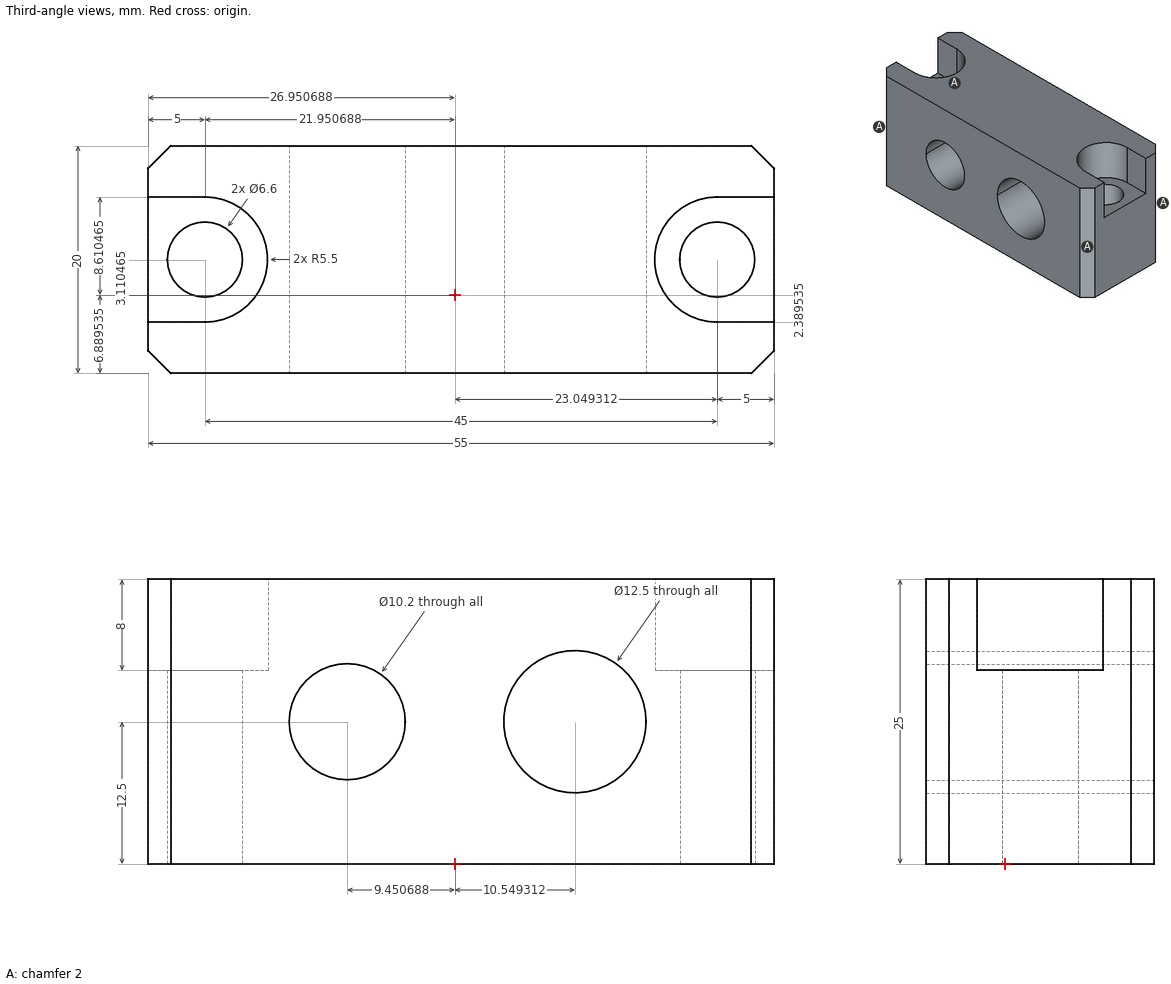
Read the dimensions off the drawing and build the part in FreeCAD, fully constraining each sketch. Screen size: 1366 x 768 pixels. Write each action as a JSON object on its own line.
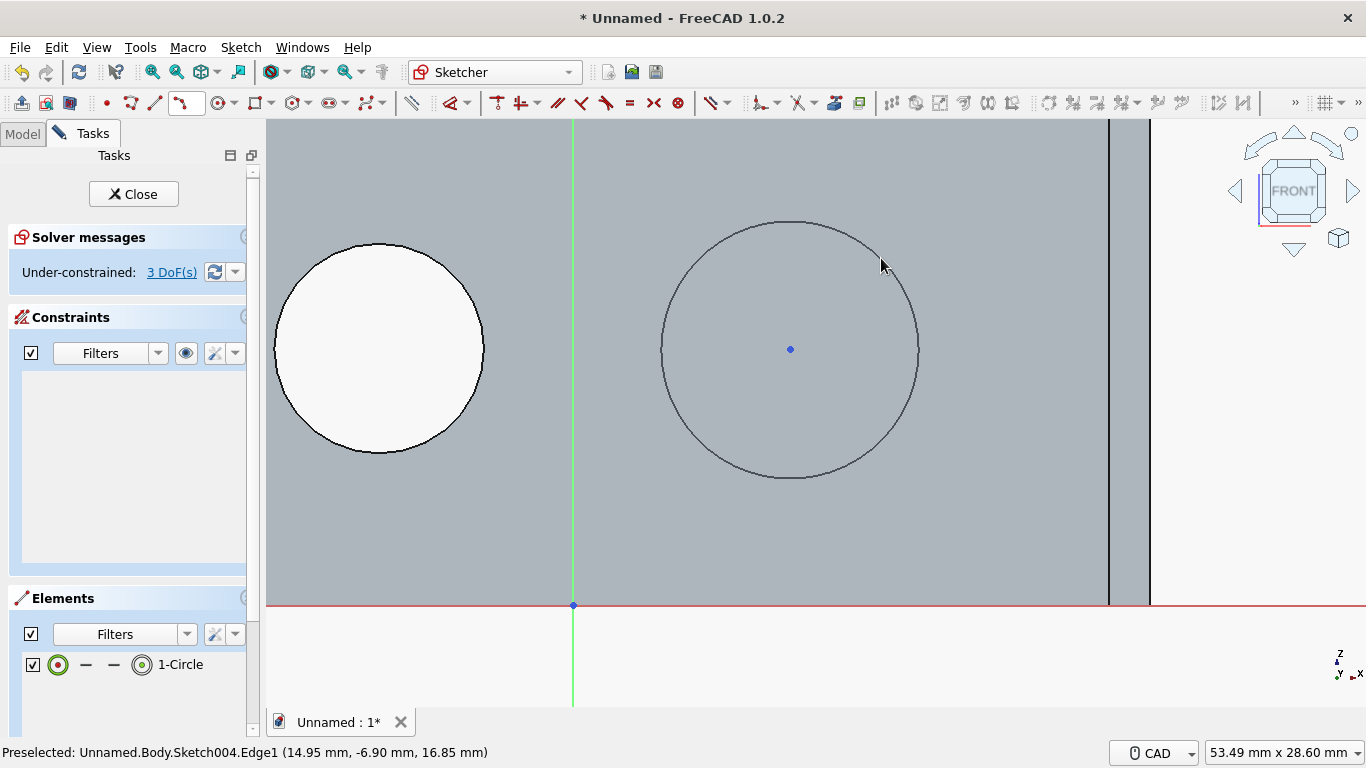
{"action": "key", "text": "d"}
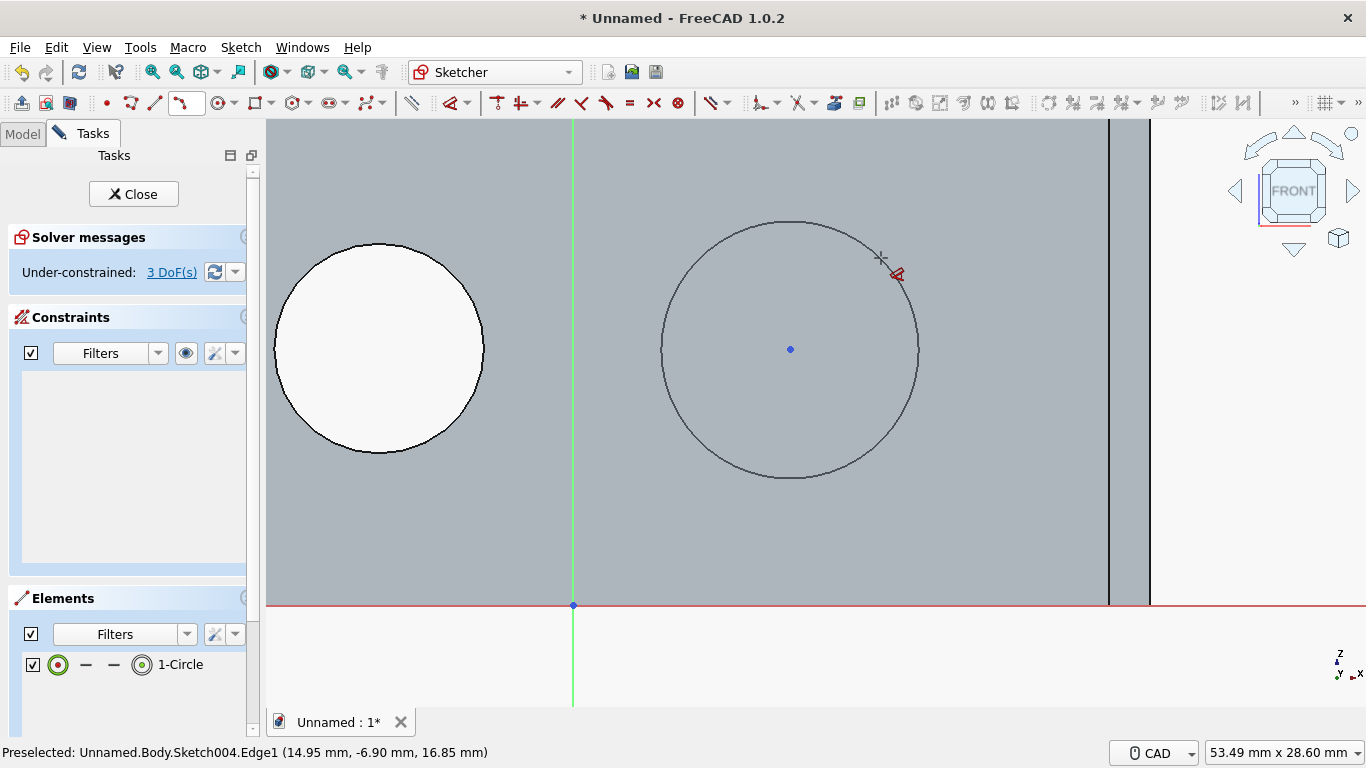
{"action": "left_click", "coordinate": [881, 259]}
{"action": "left_click", "coordinate": [904, 236]}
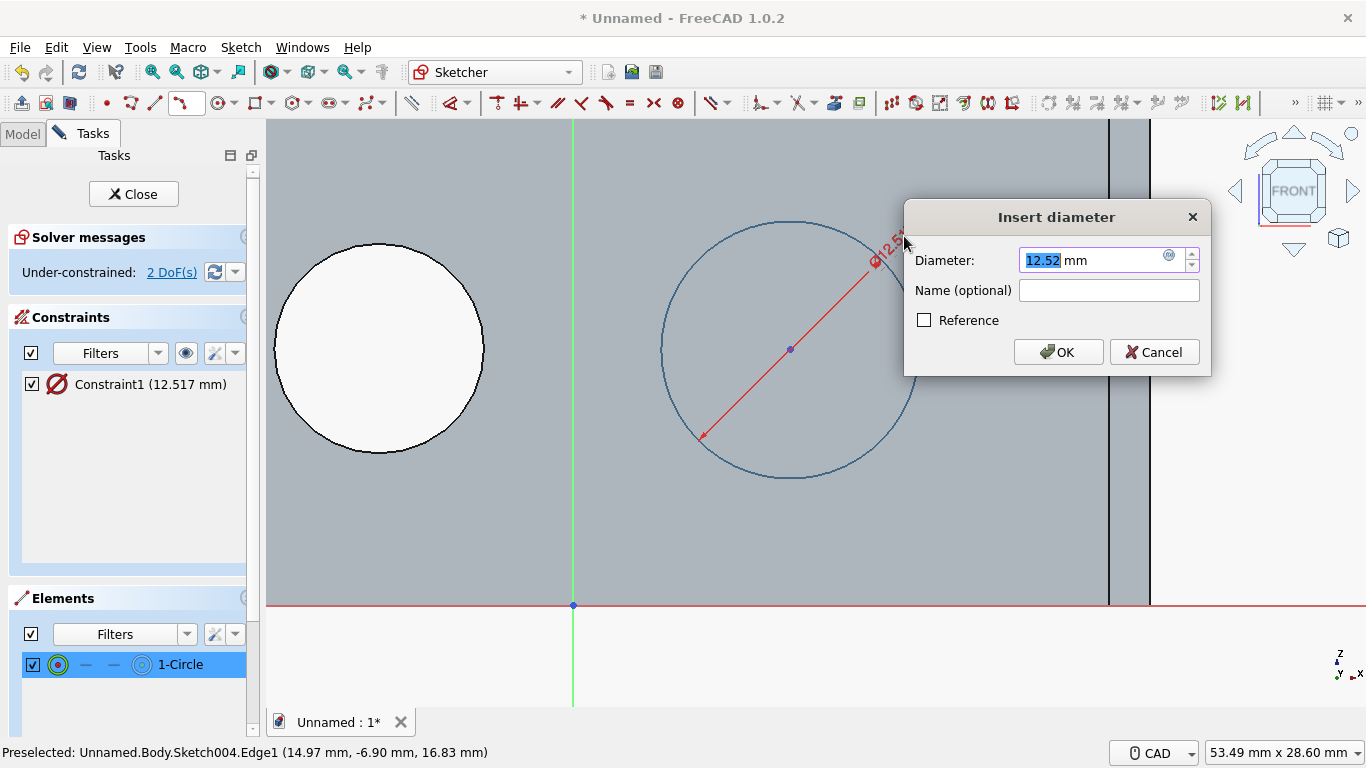
{"action": "type", "text": "12.5"}
{"action": "key", "text": "Return"}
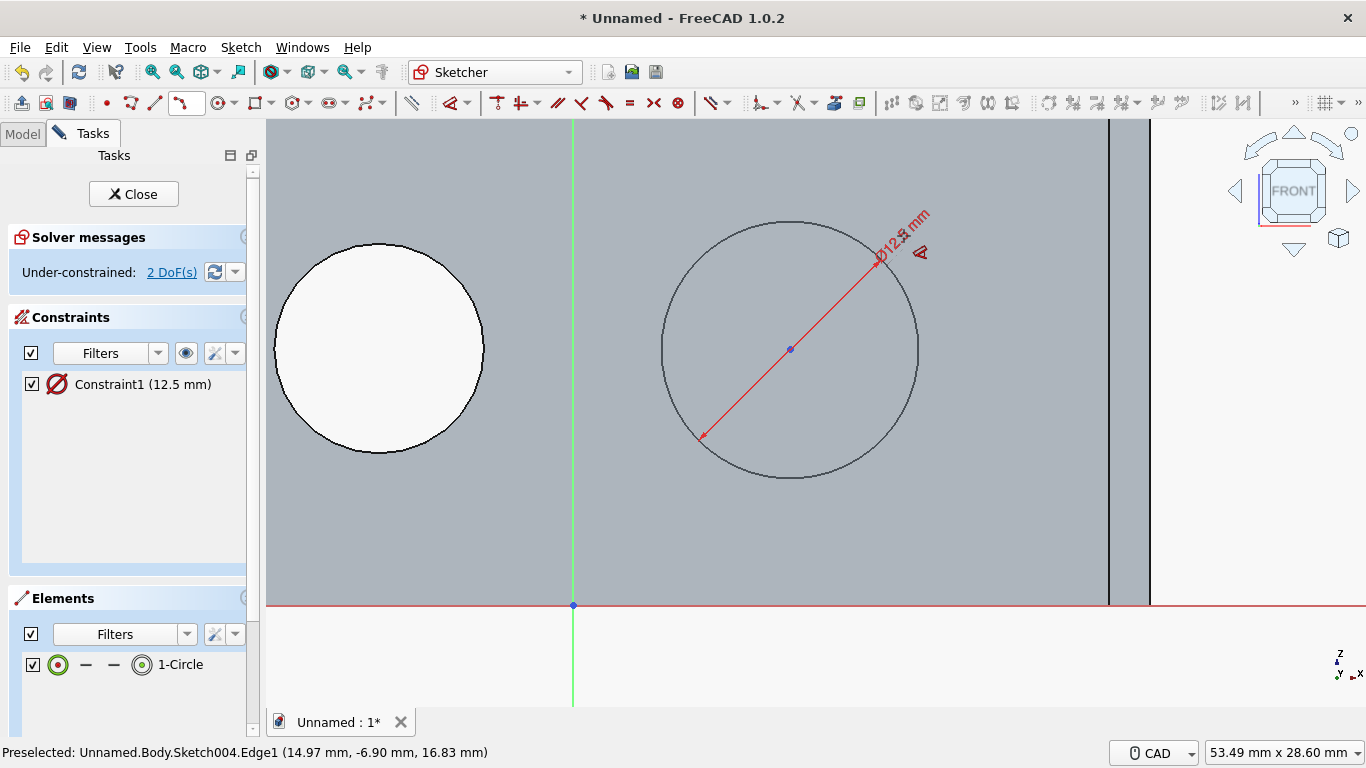
{"action": "left_click", "coordinate": [790, 350]}
{"action": "left_click", "coordinate": [539, 478]}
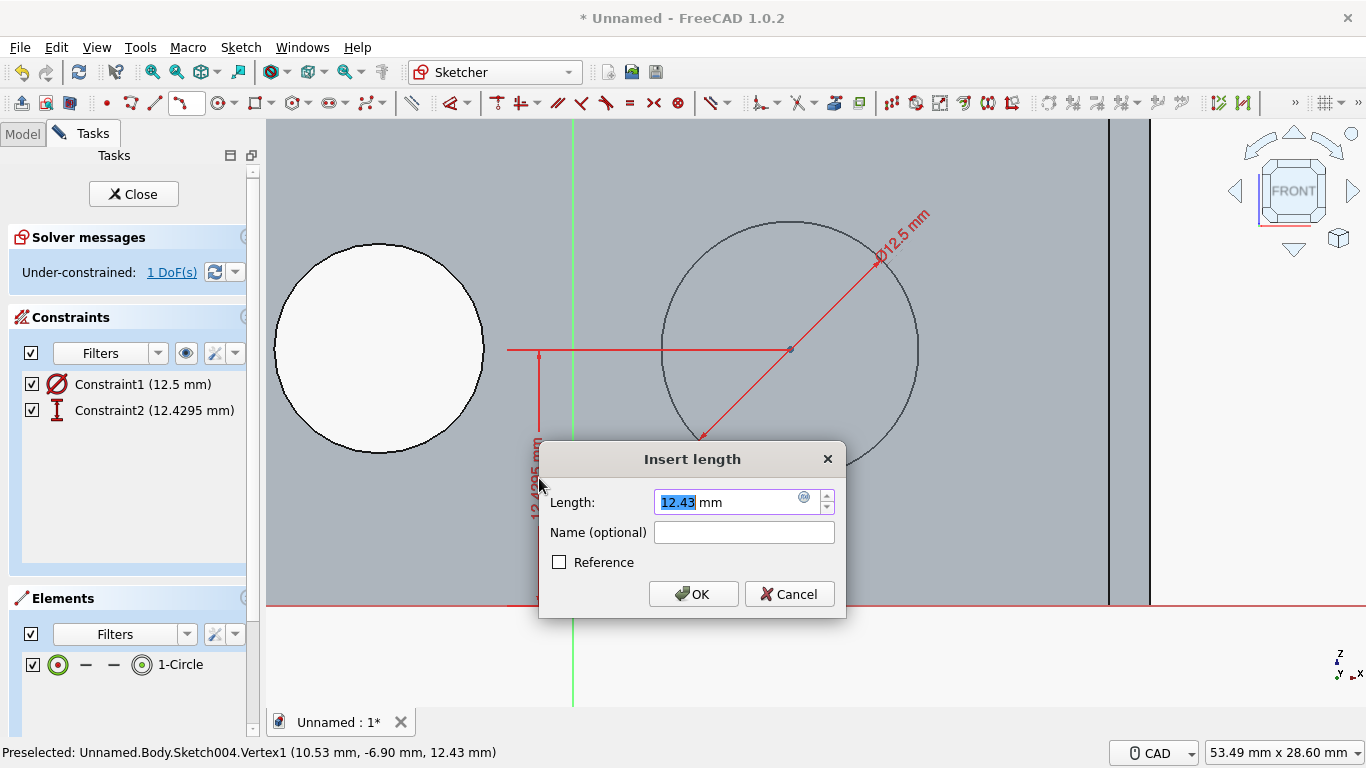
{"action": "type", "text": "12.5"}
{"action": "key", "text": "Return"}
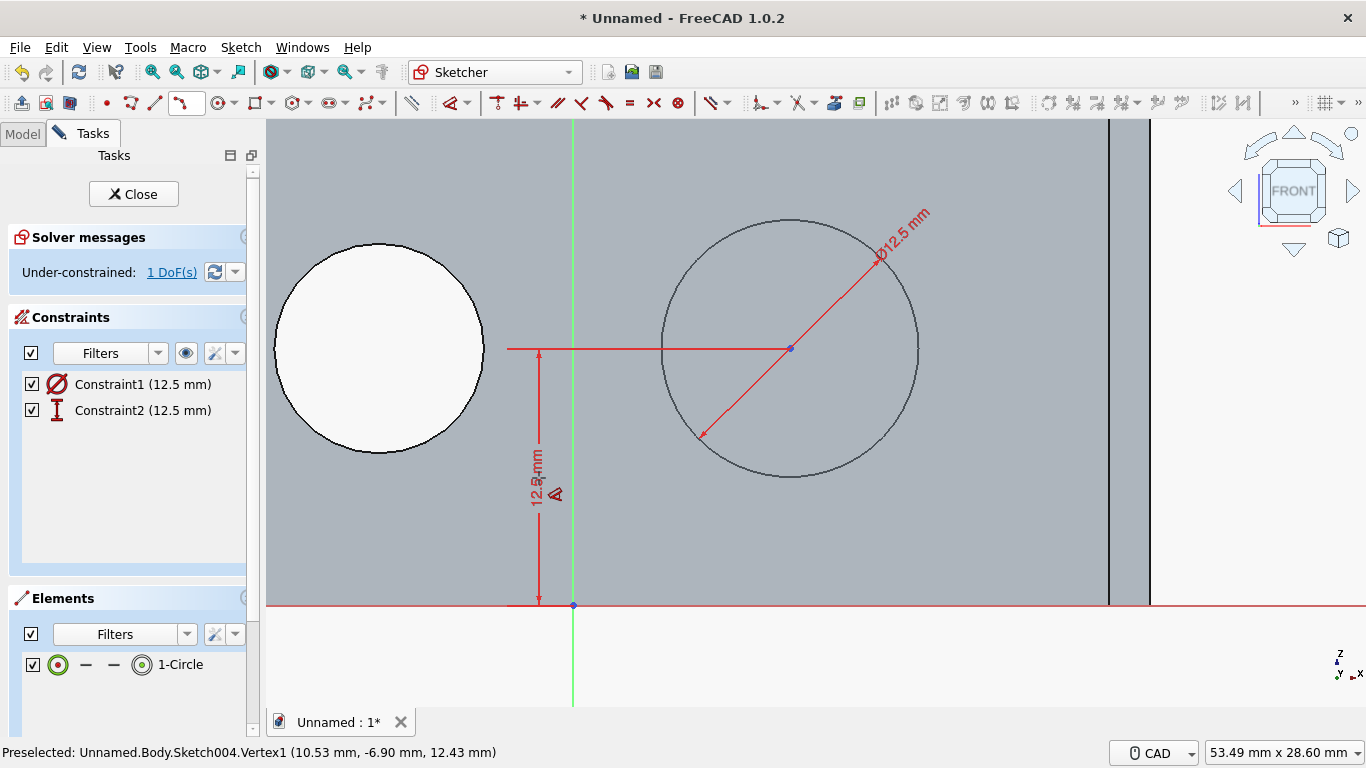
{"action": "left_click", "coordinate": [790, 349]}
{"action": "left_click", "coordinate": [682, 640]}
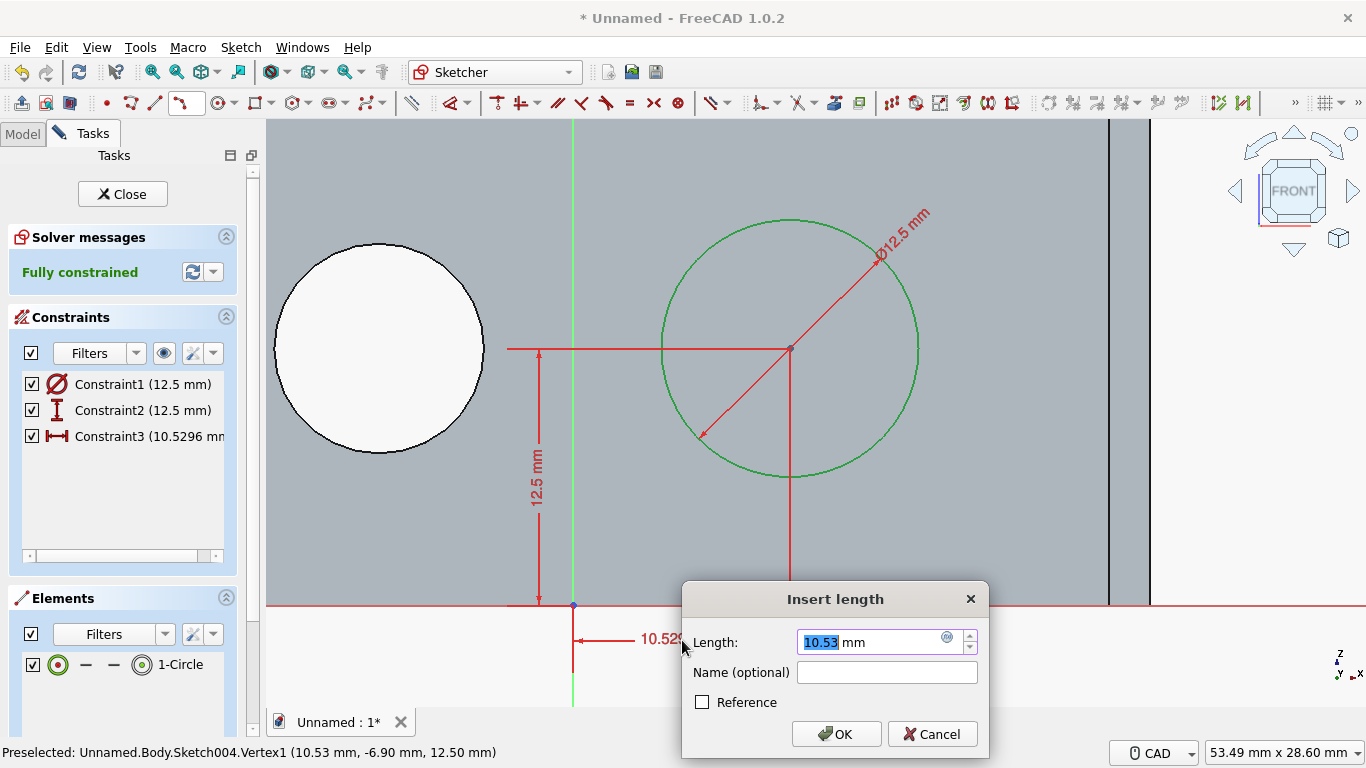
{"action": "type", "text": "10.549312"}
{"action": "key", "text": "Return"}
{"action": "key", "text": "Escape"}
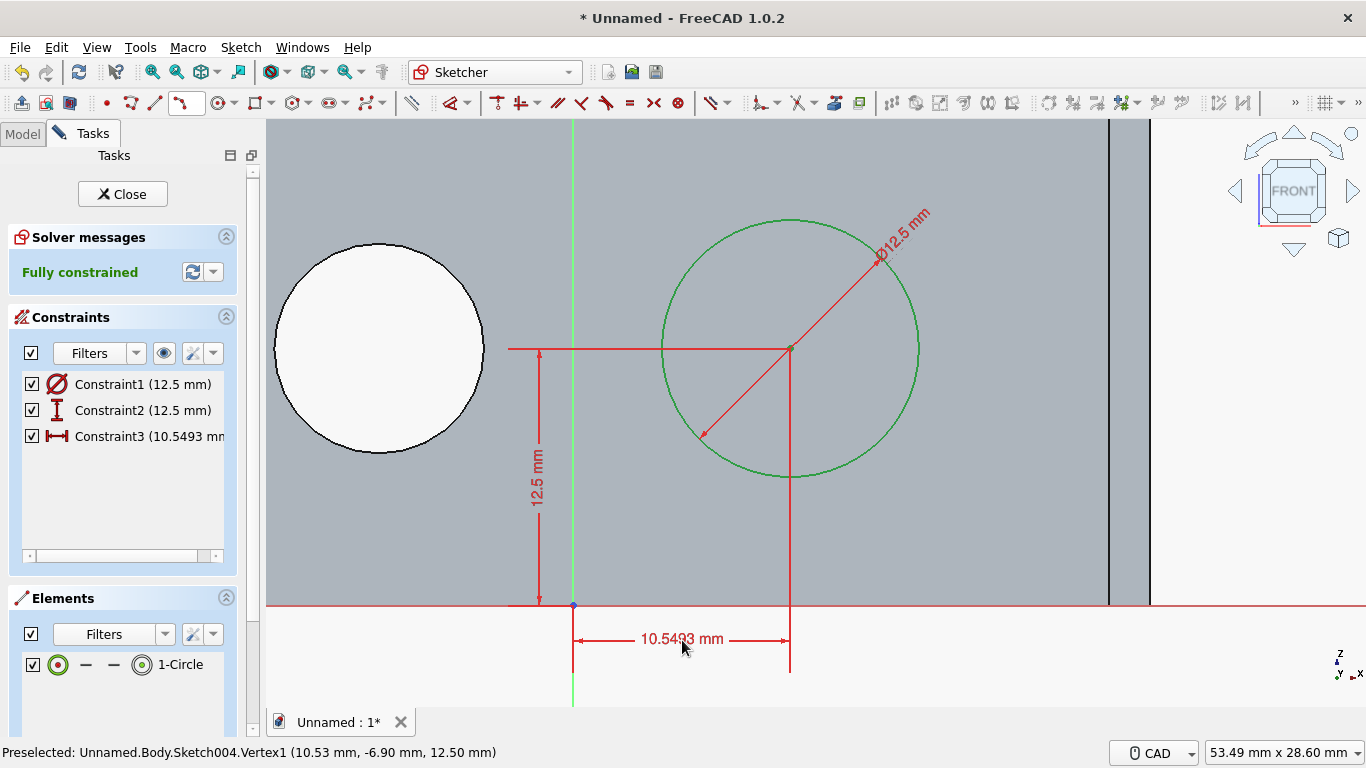
{"action": "left_click", "coordinate": [123, 194]}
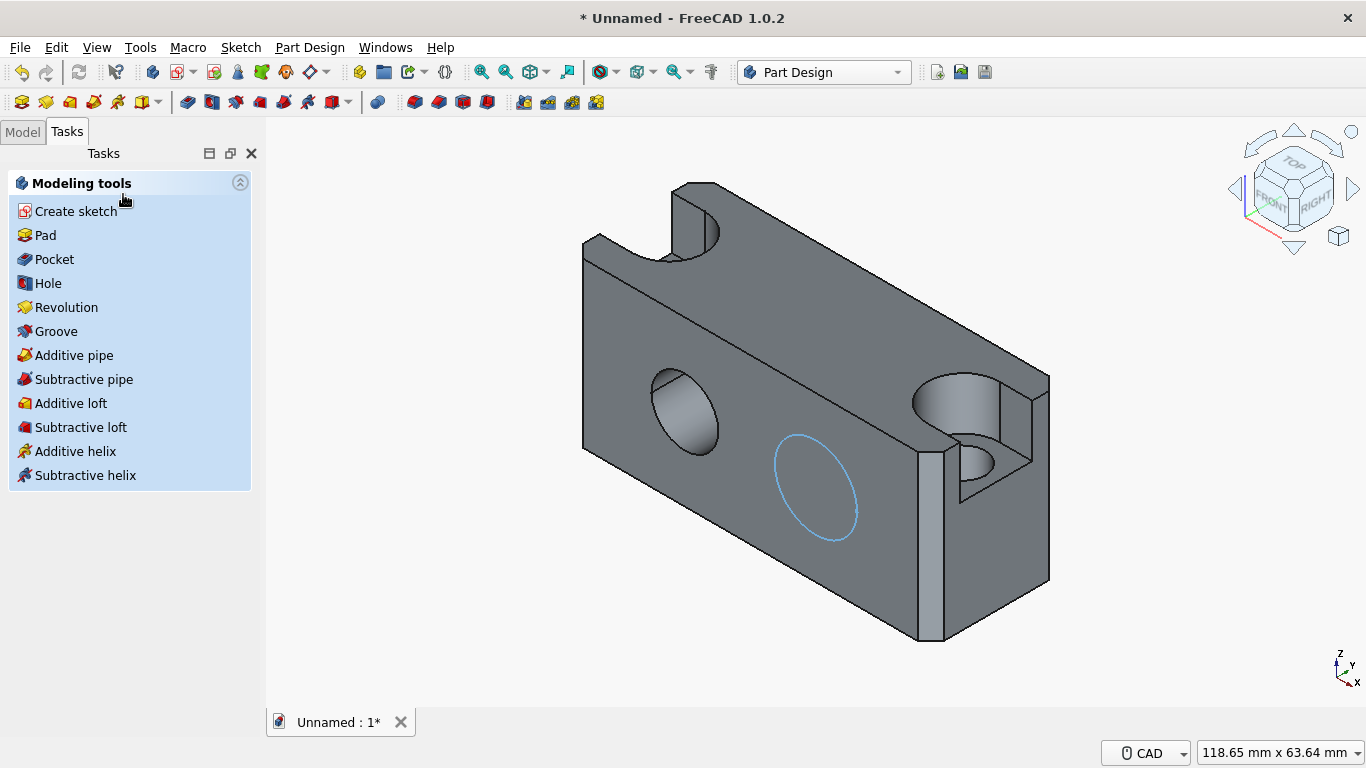
{"action": "left_click", "coordinate": [212, 102]}